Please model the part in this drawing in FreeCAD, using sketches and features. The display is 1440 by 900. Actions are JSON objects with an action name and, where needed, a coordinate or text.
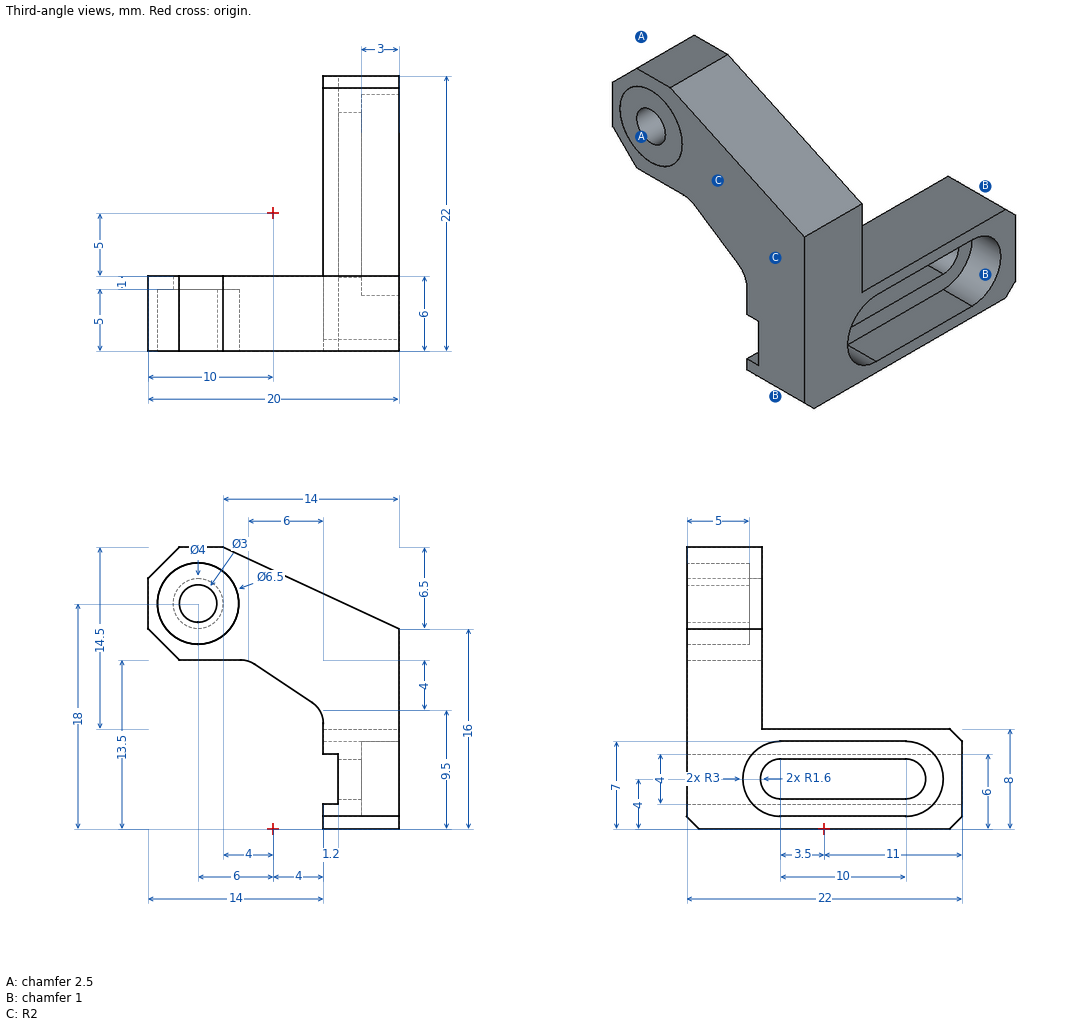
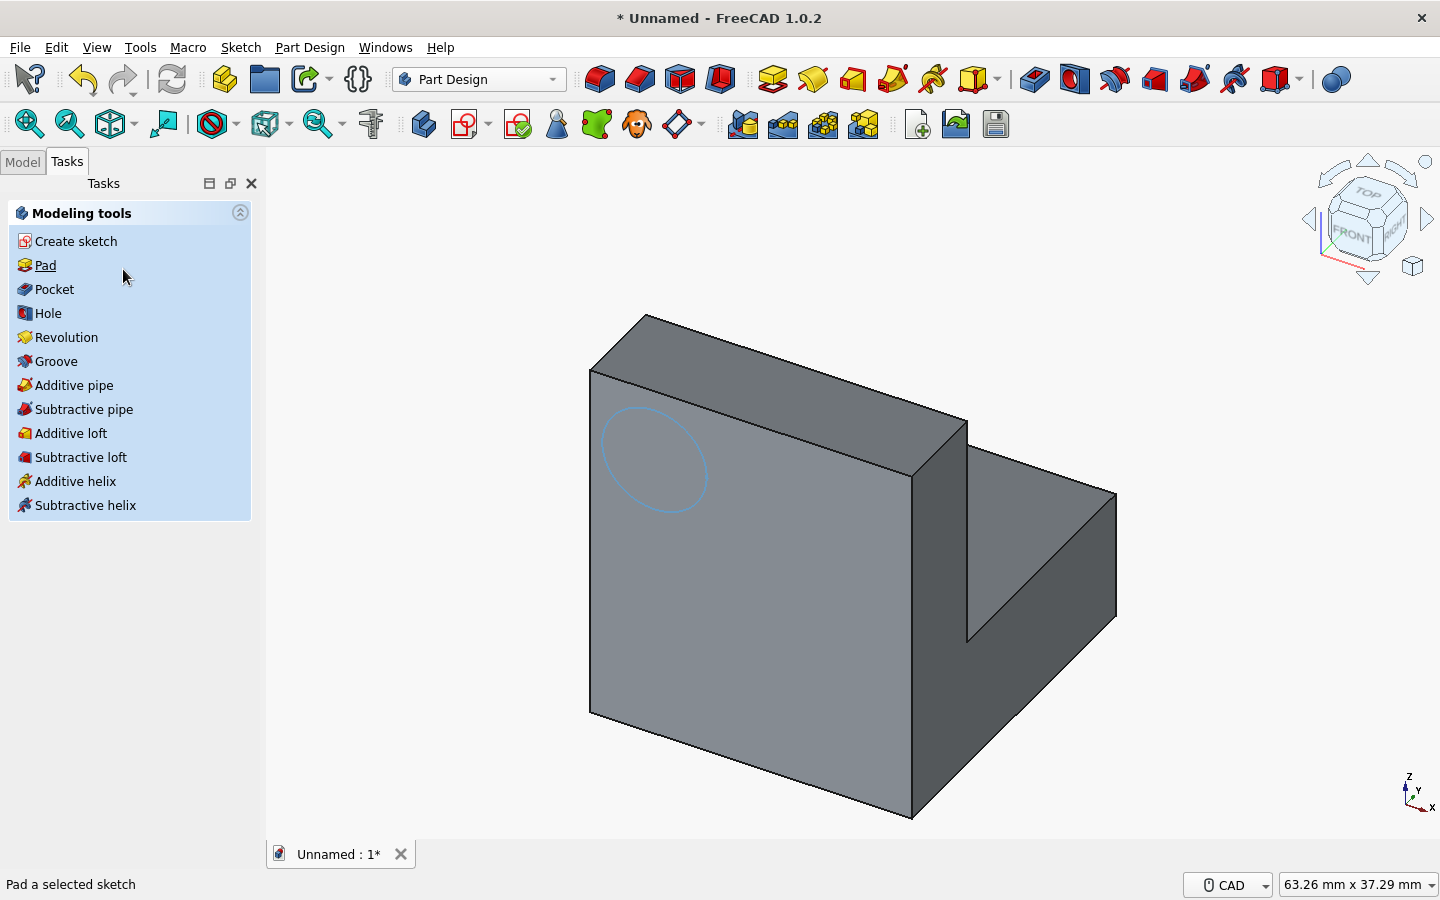
{"action": "left_click", "coordinate": [1036, 80]}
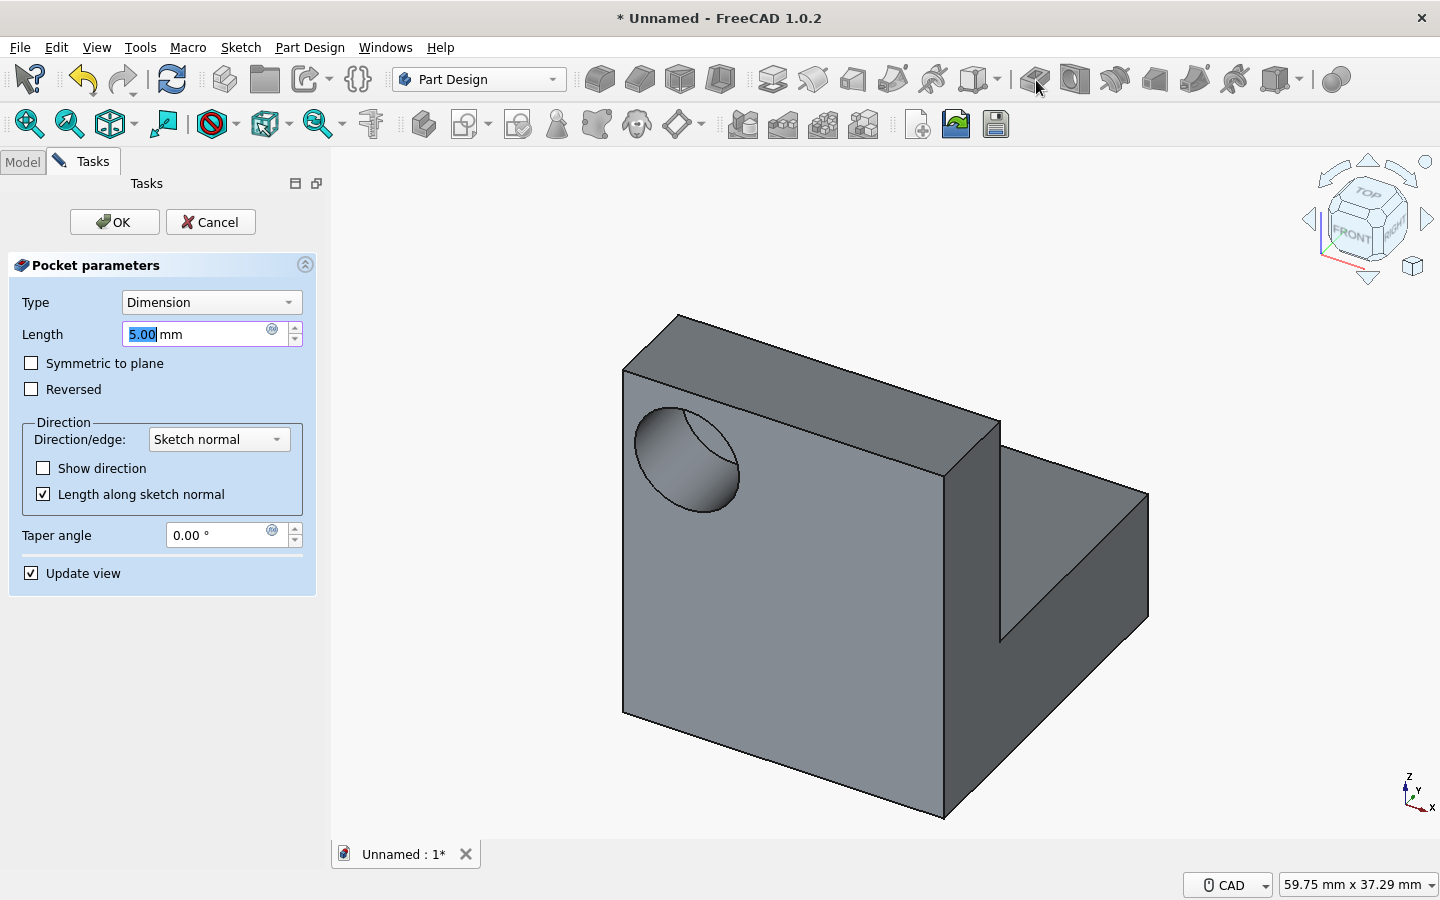
{"action": "type", "text": "5"}
{"action": "key", "text": "Tab"}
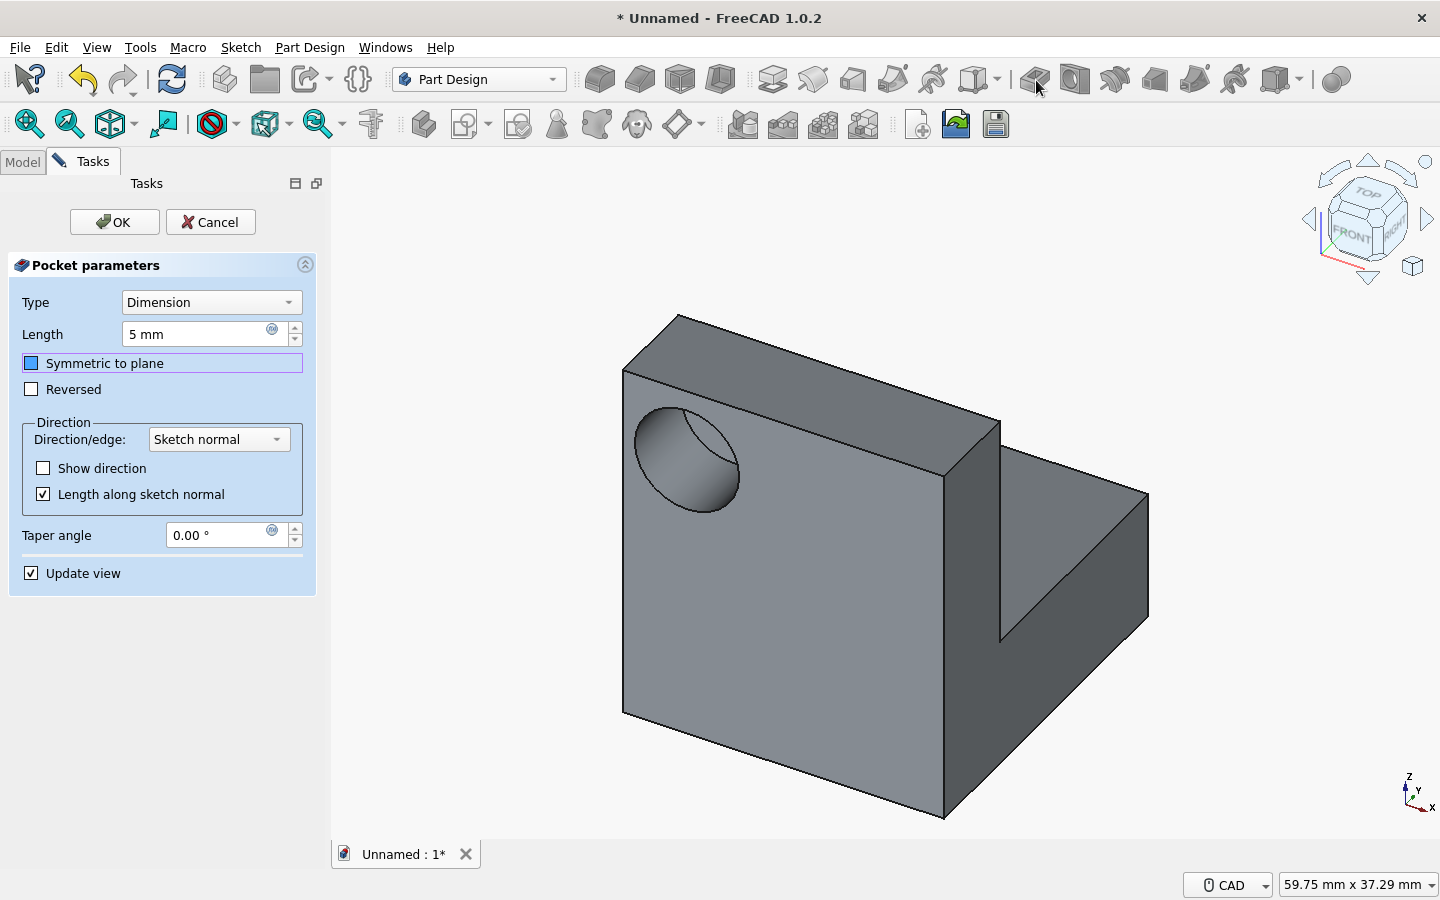
{"action": "left_click", "coordinate": [115, 222]}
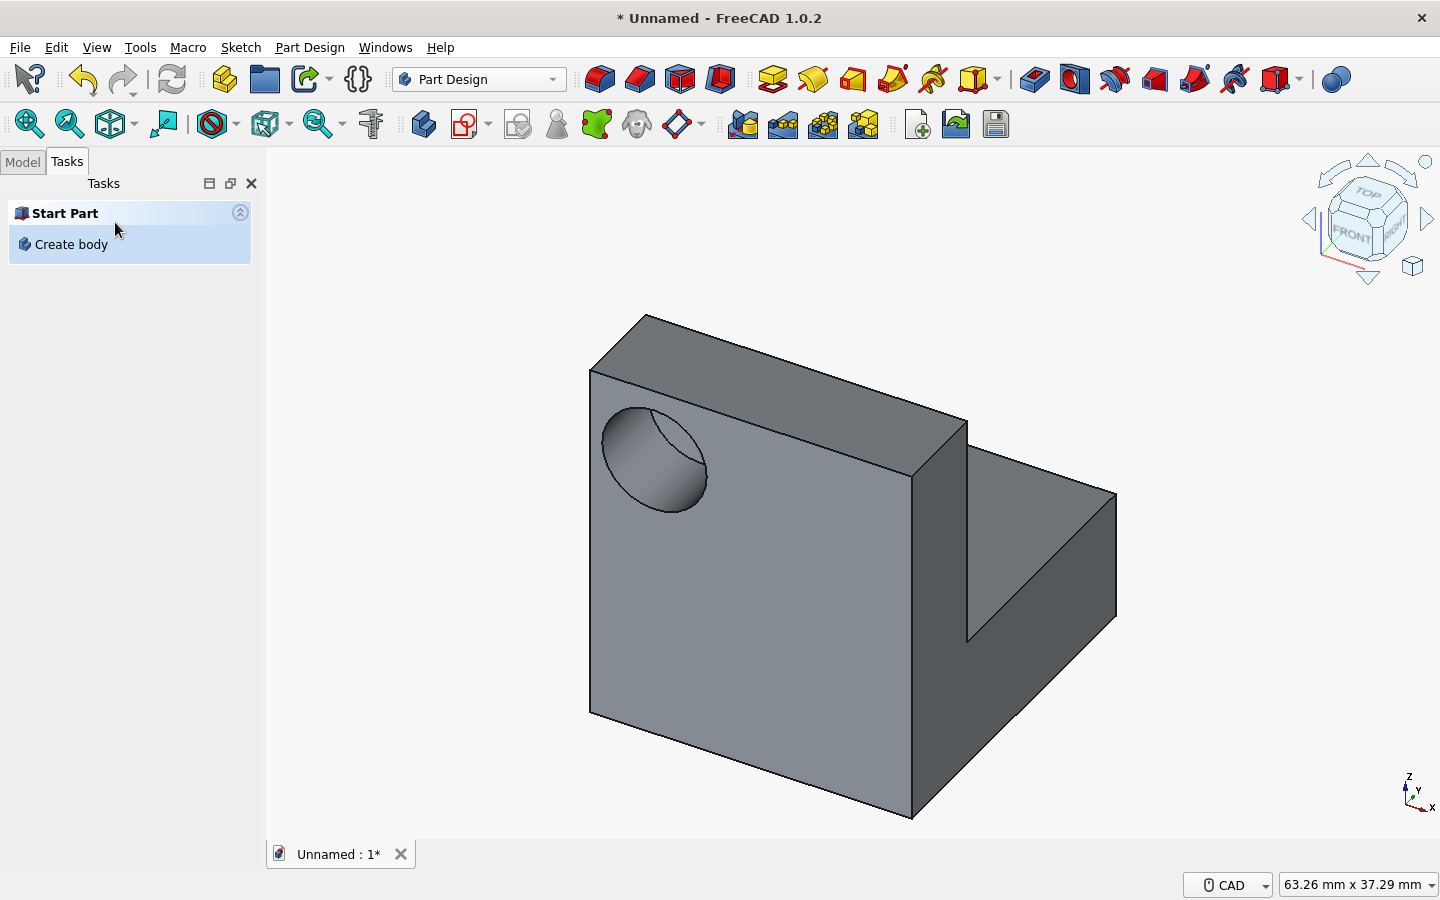
{"action": "left_click", "coordinate": [751, 642]}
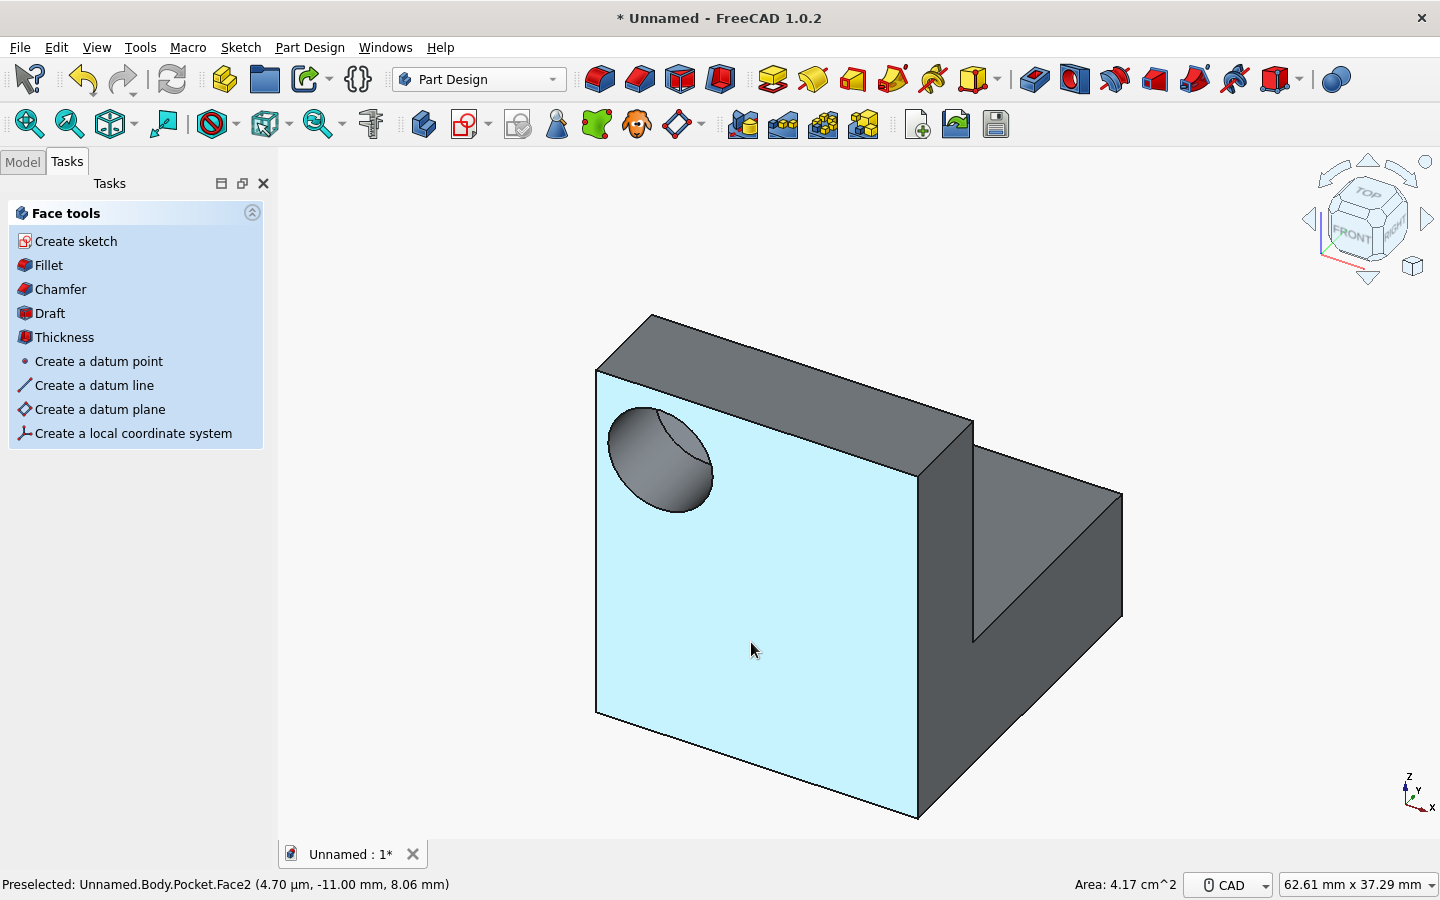
{"action": "left_click", "coordinate": [464, 124]}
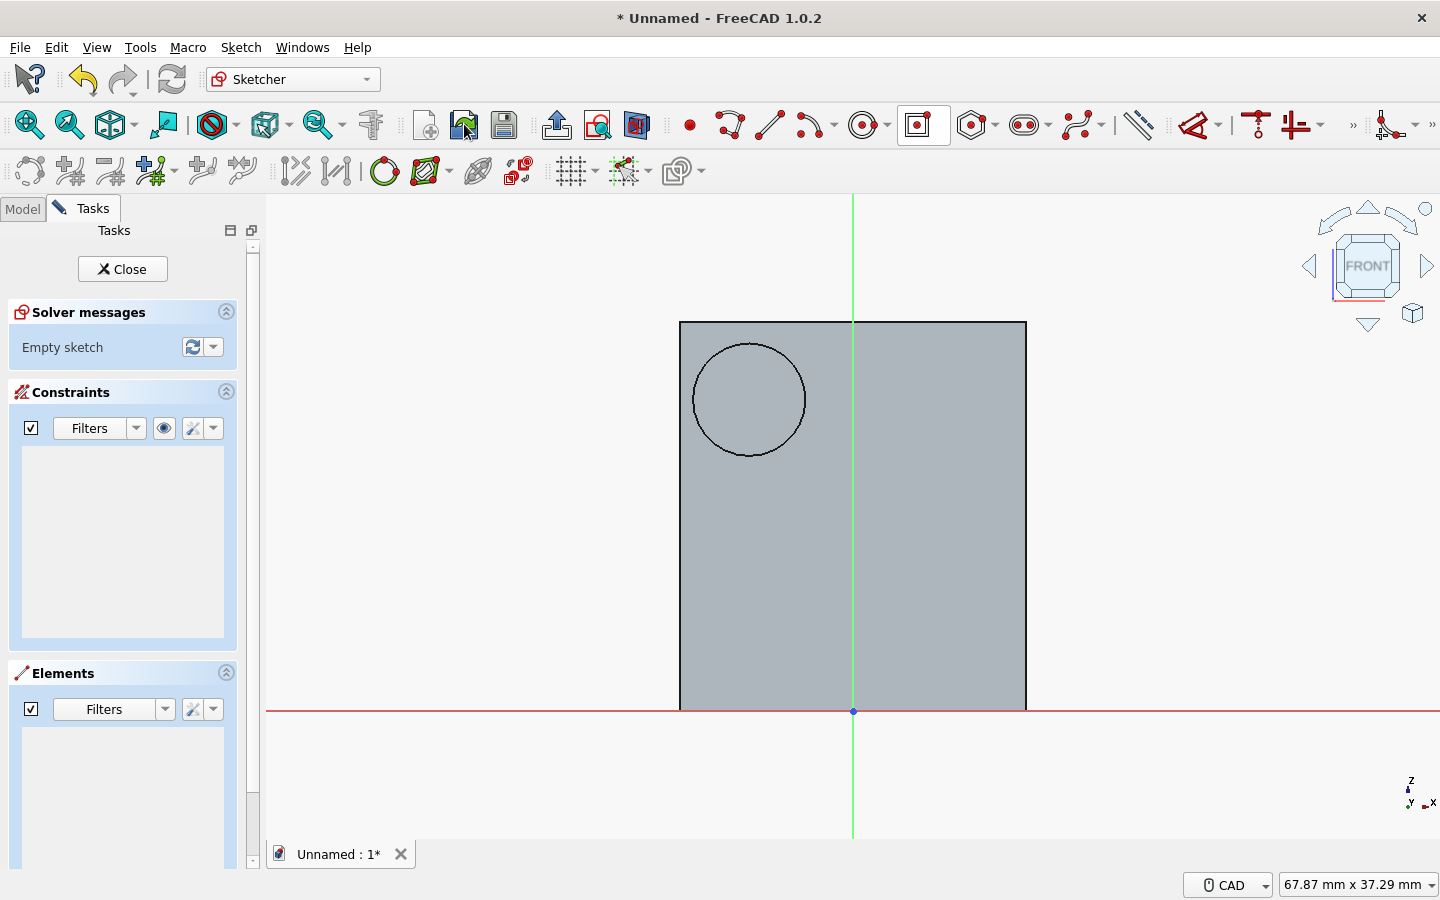
{"action": "scroll", "coordinate": [821, 689], "scroll_direction": "up", "scroll_amount": 3}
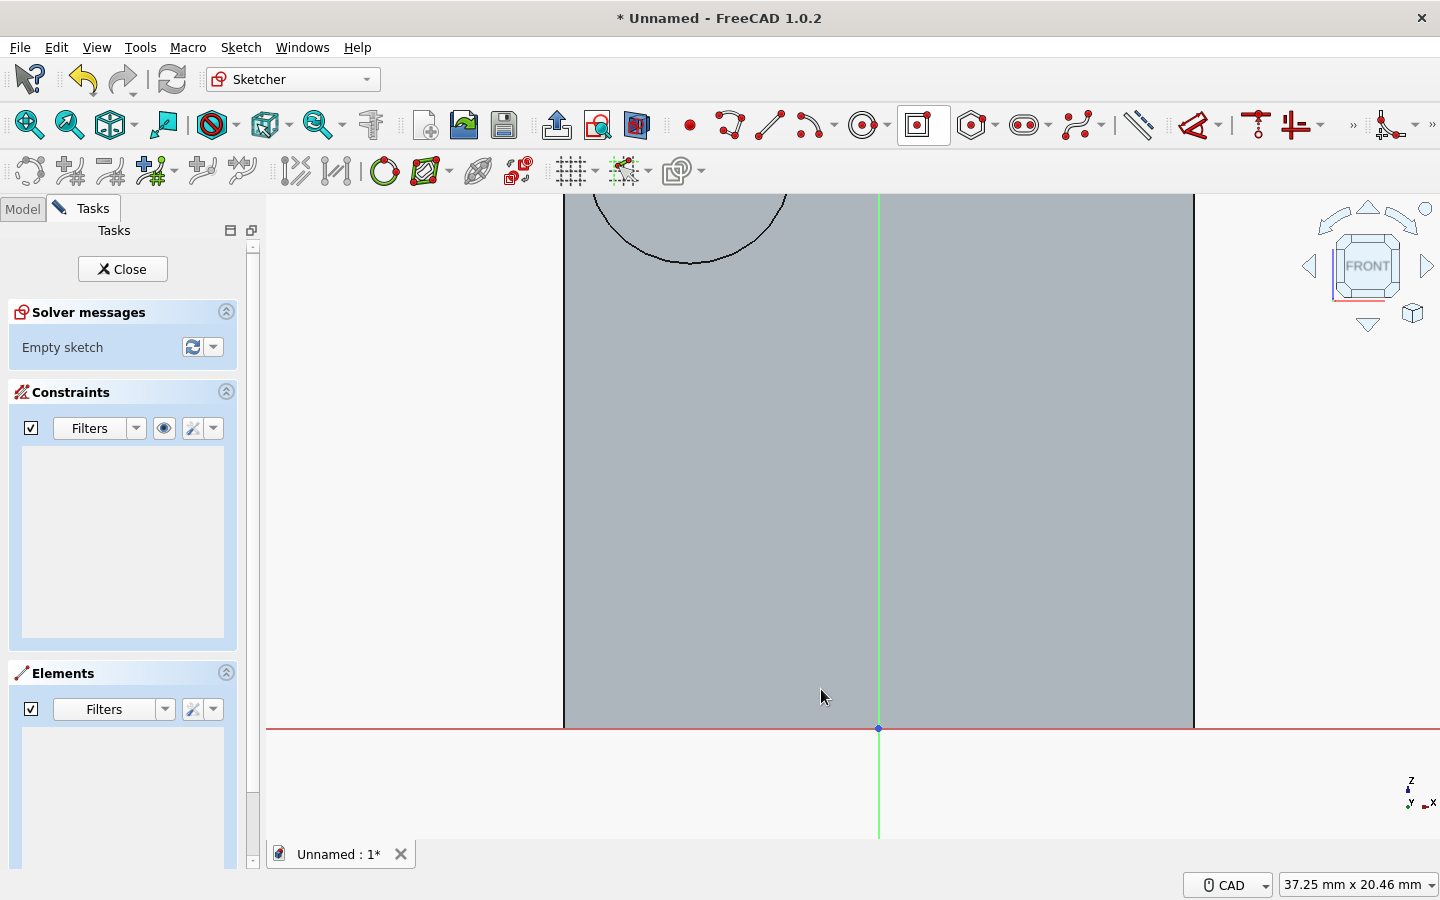
{"action": "key", "text": "g r"}